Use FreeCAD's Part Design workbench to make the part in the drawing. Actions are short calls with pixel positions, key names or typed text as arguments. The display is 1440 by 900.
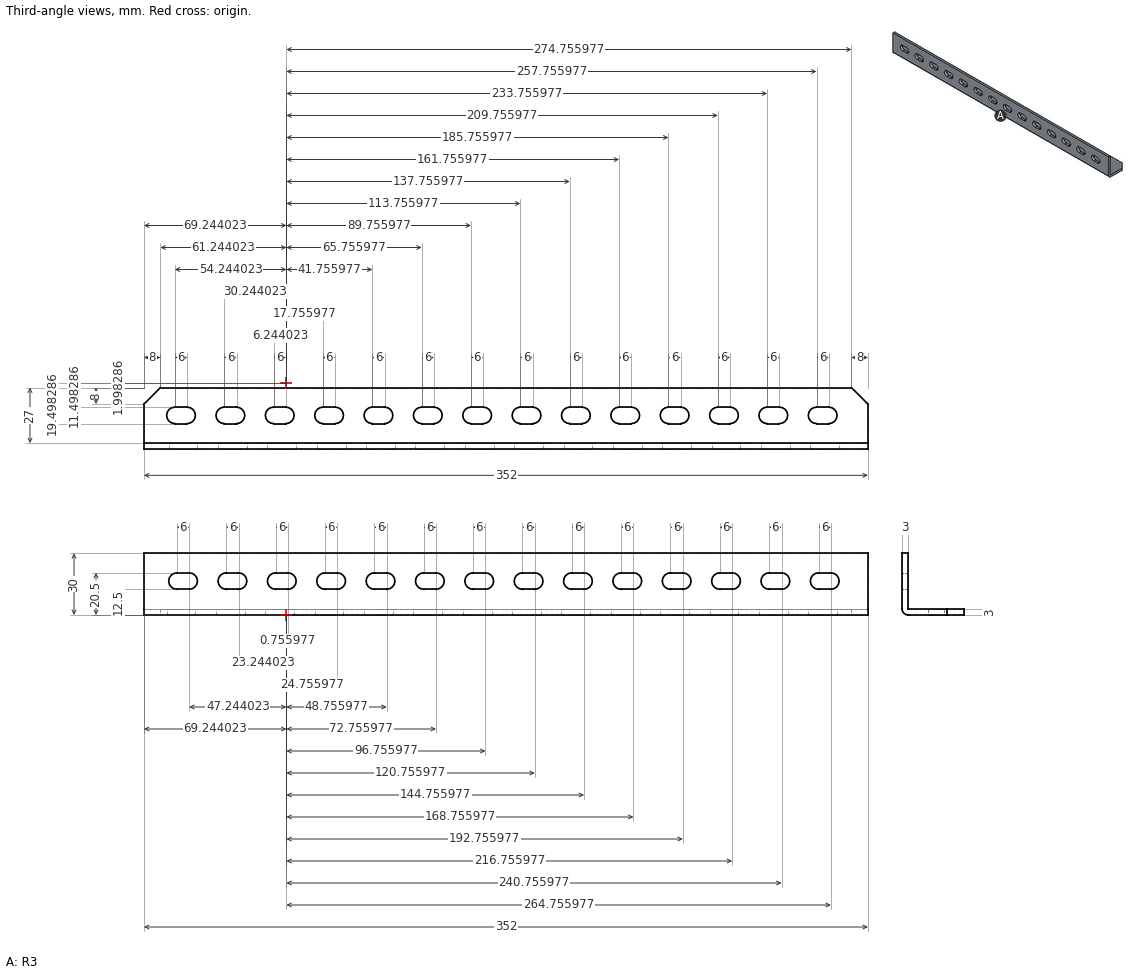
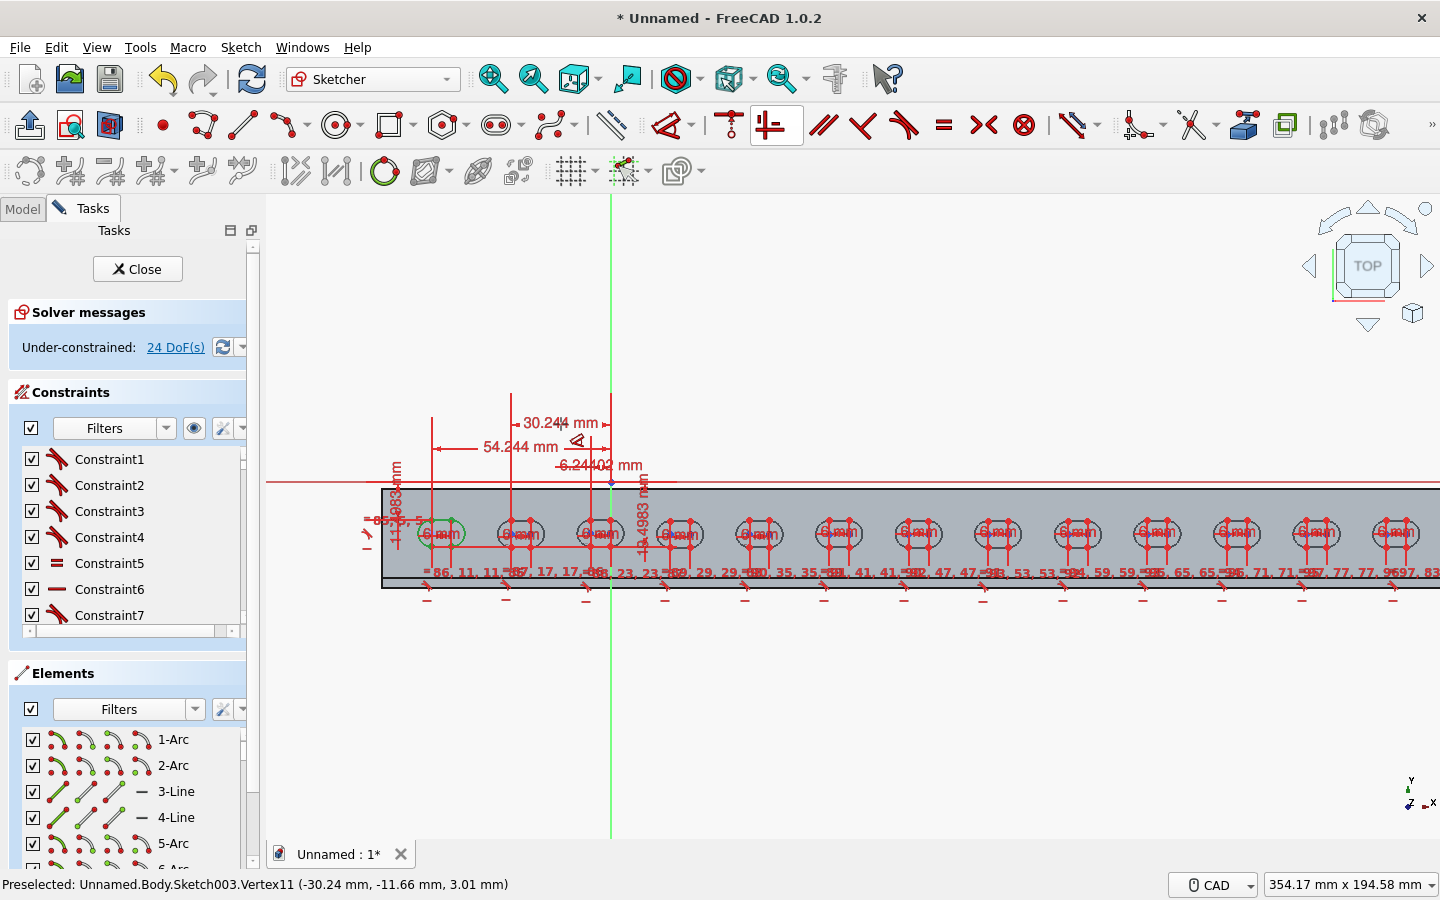
click(511, 521)
click(477, 501)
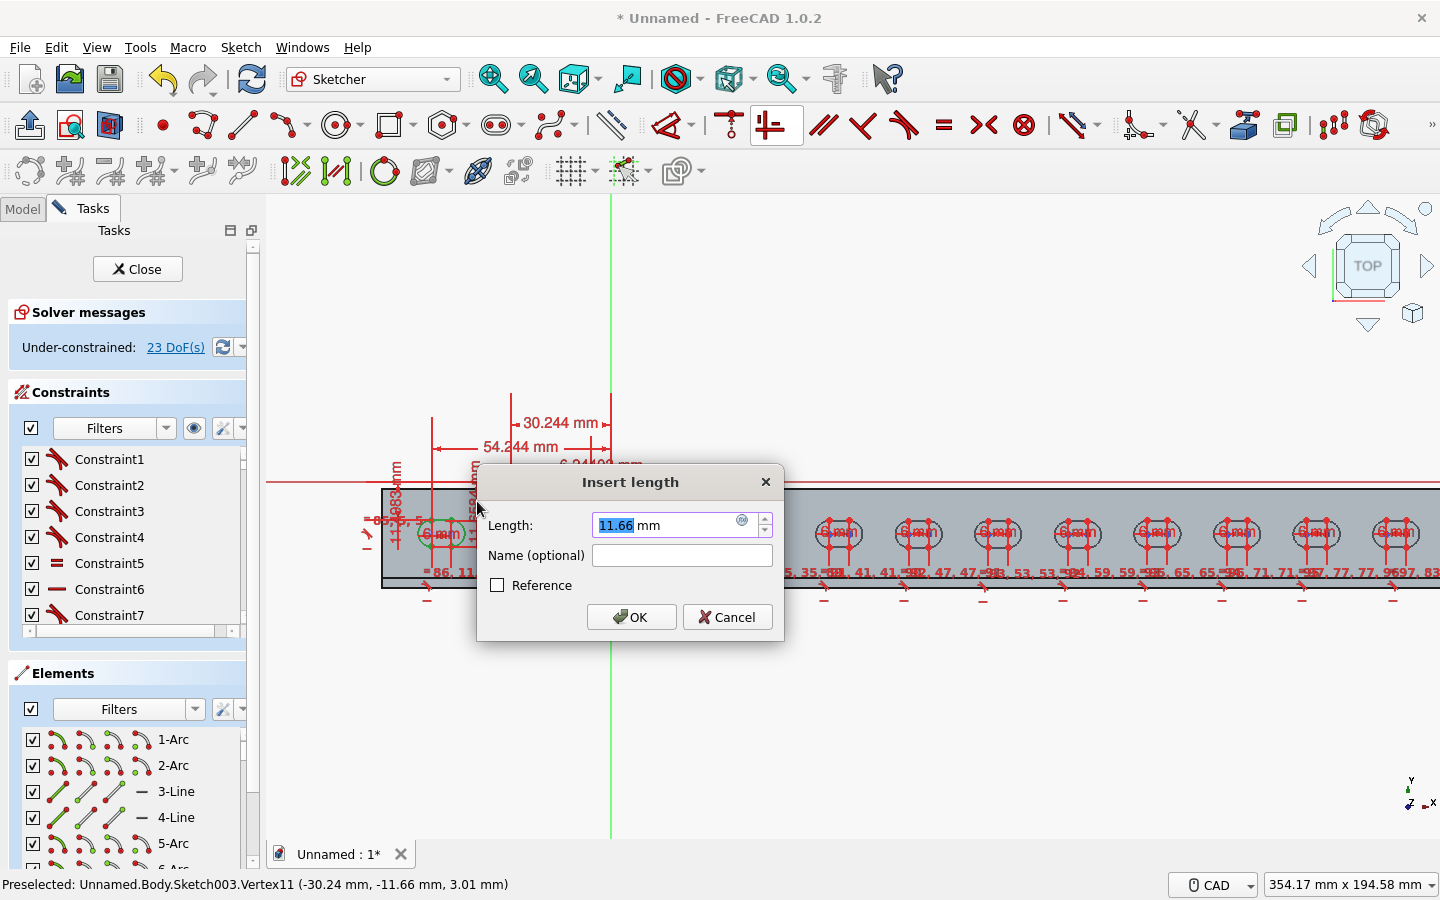
text(11.498286)
key(Return)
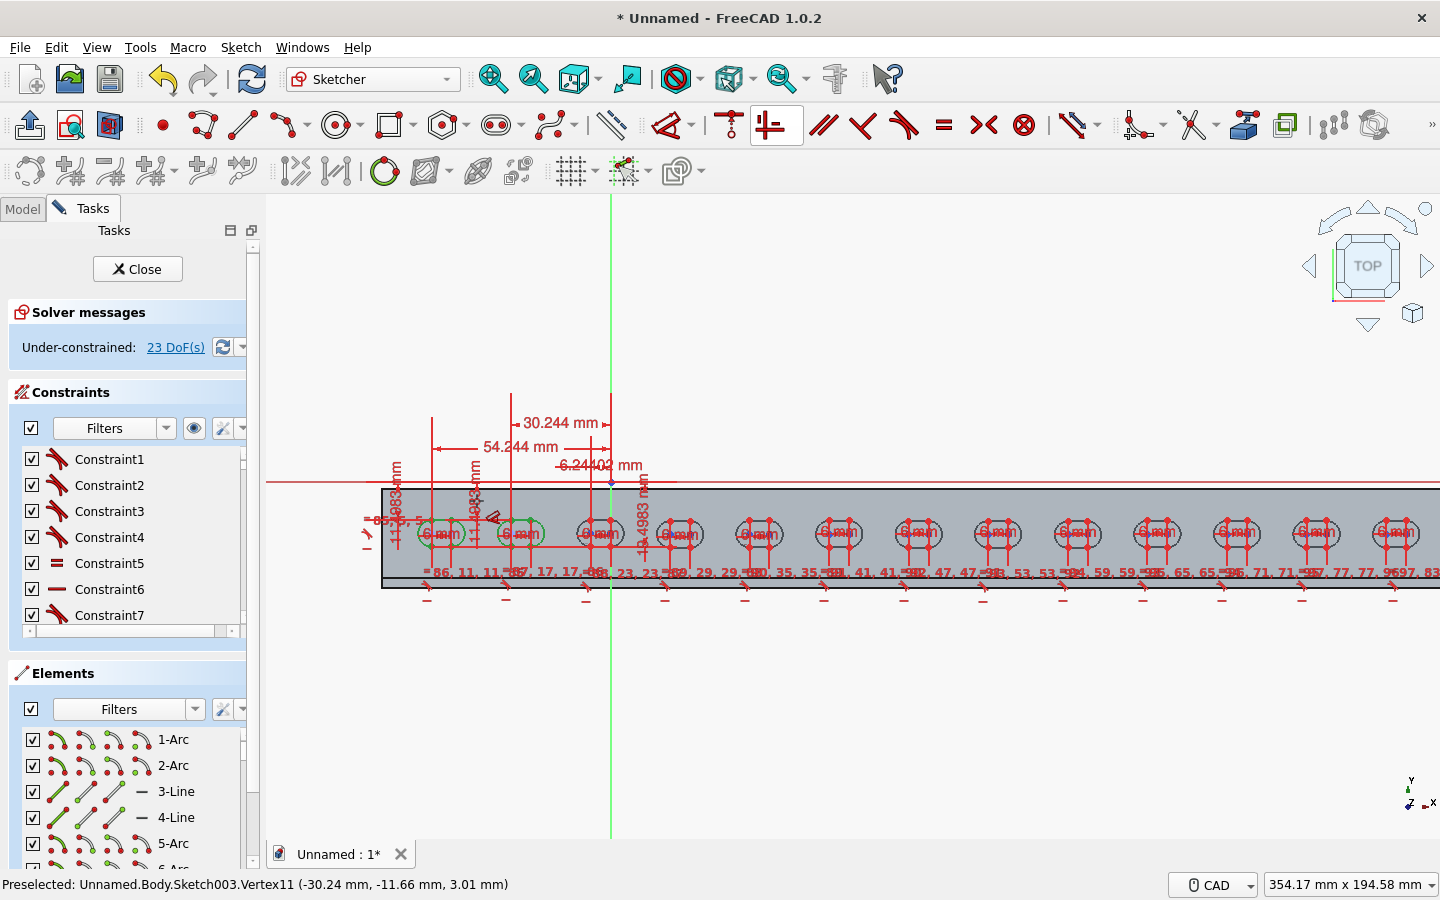
click(591, 520)
click(557, 501)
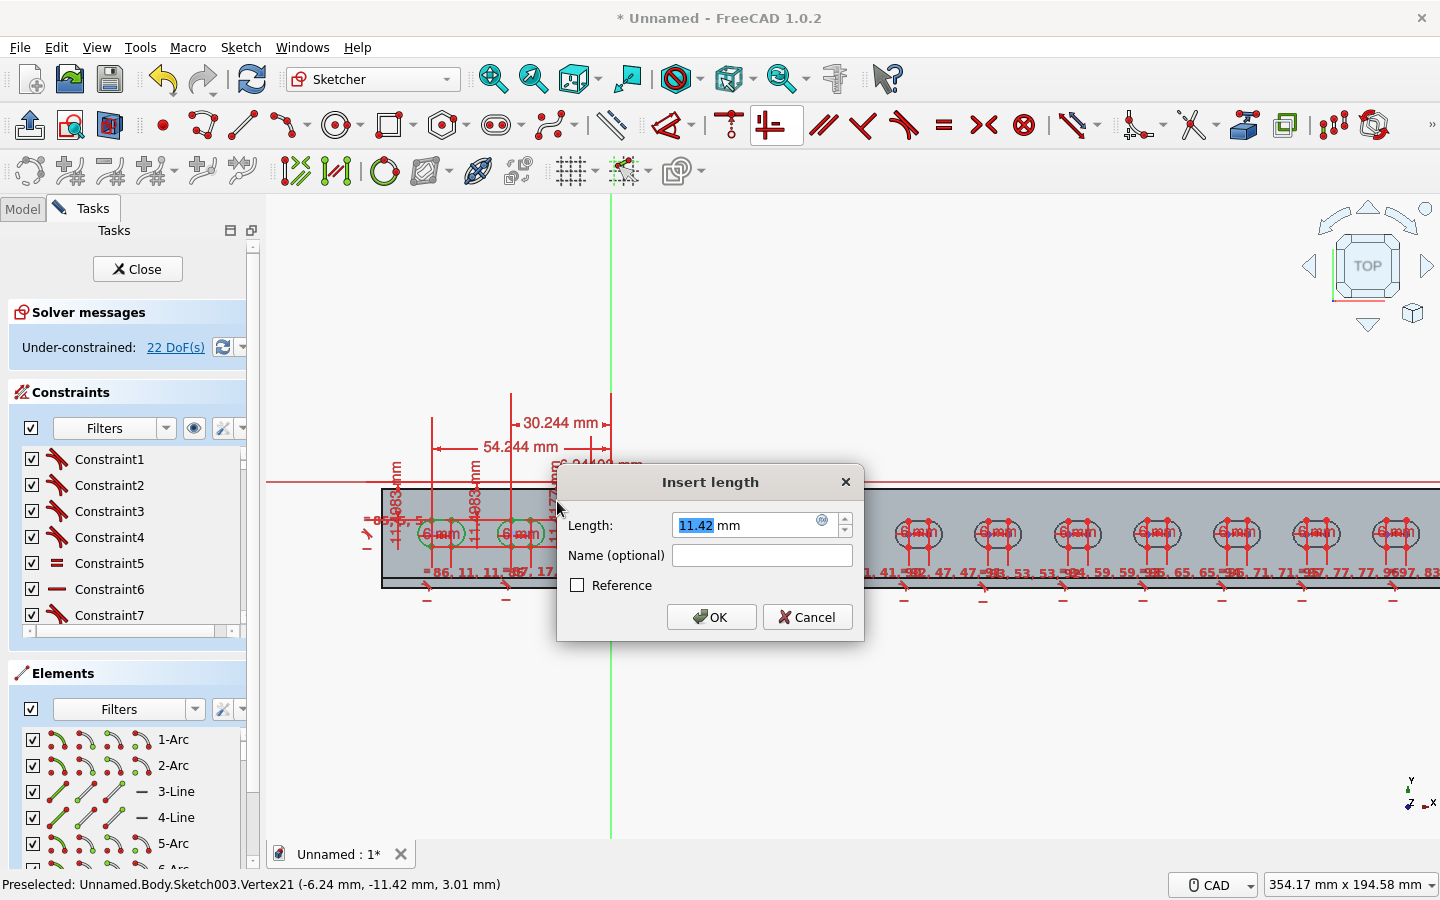
text(11.498286)
key(Return)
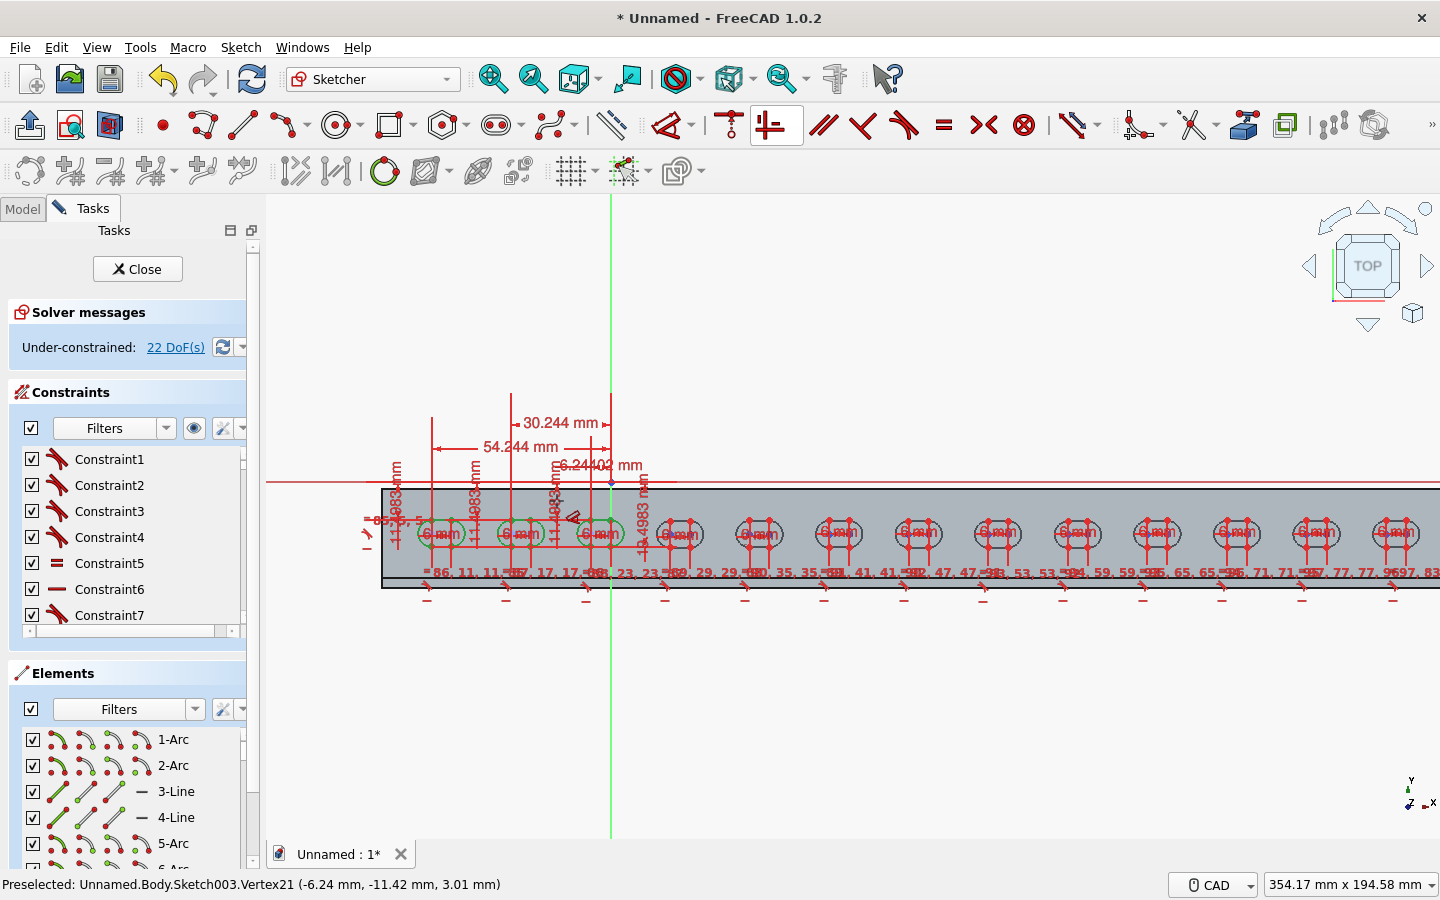
click(670, 521)
click(641, 424)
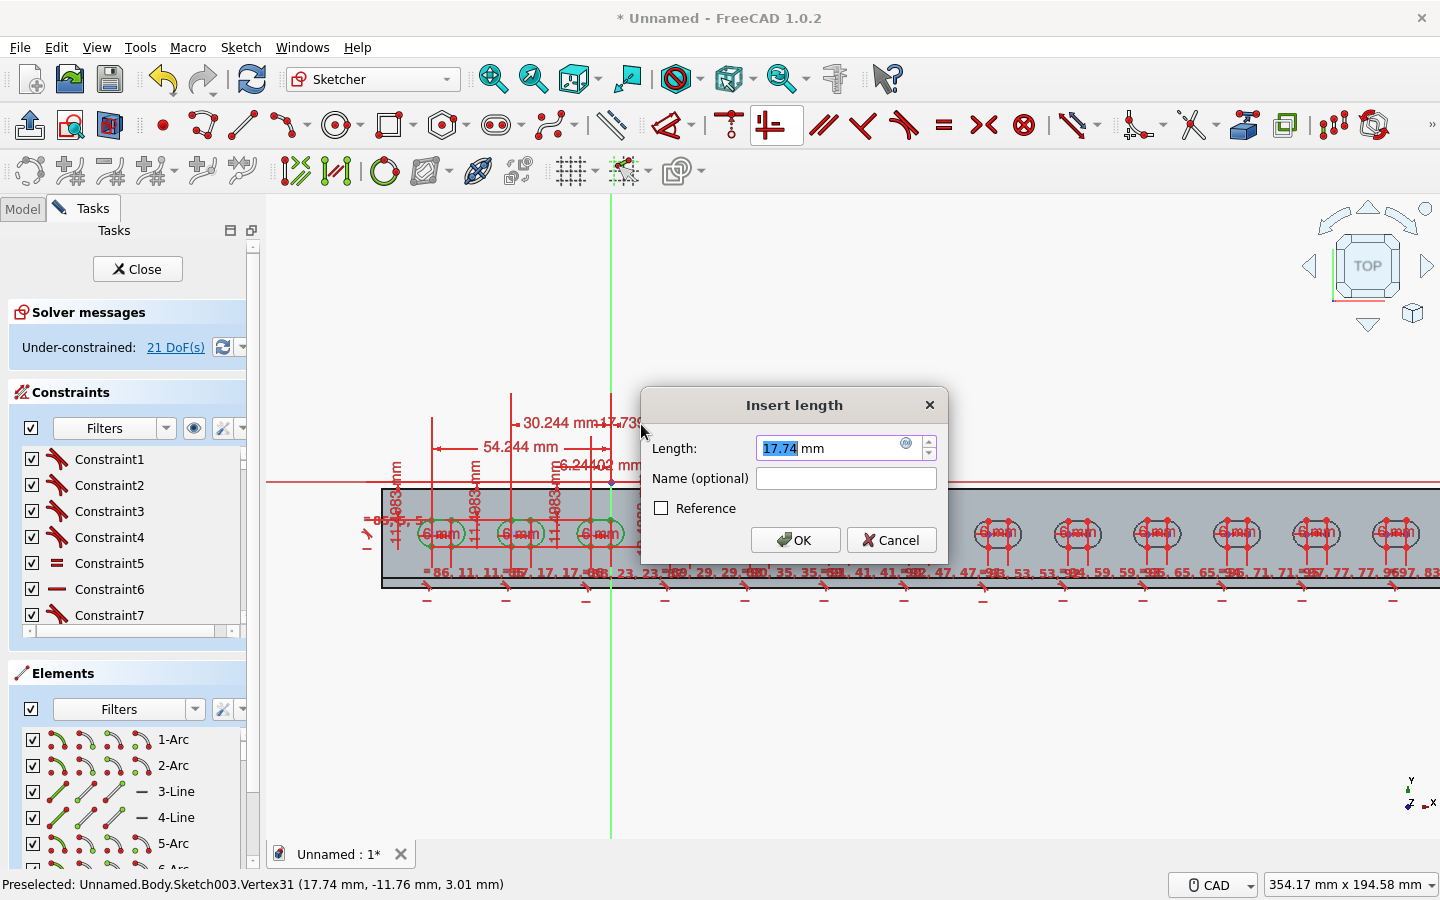
text(17.755977)
key(Return)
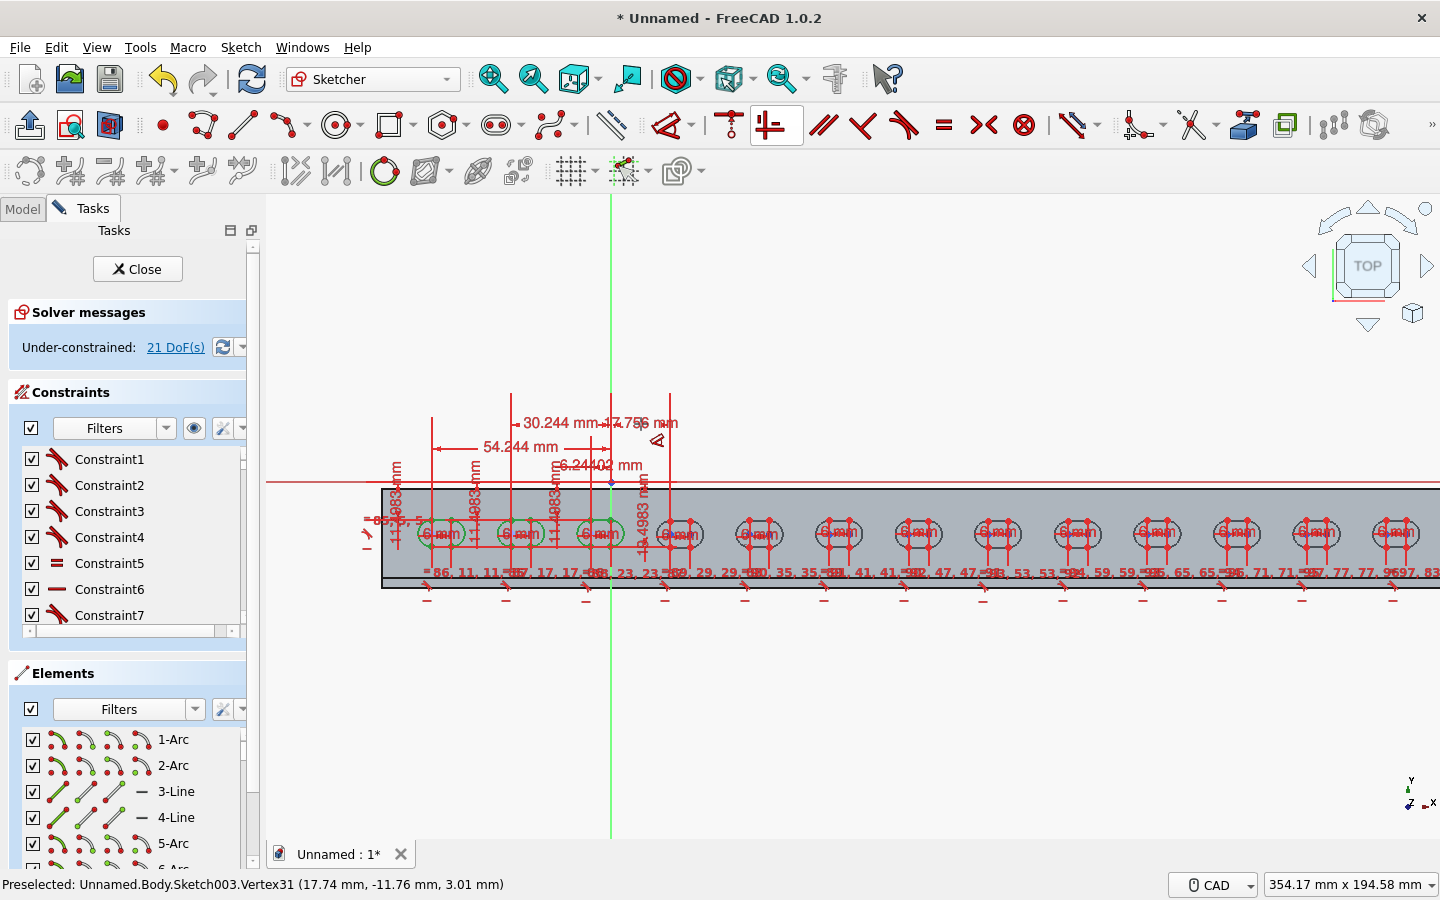
click(670, 521)
click(728, 502)